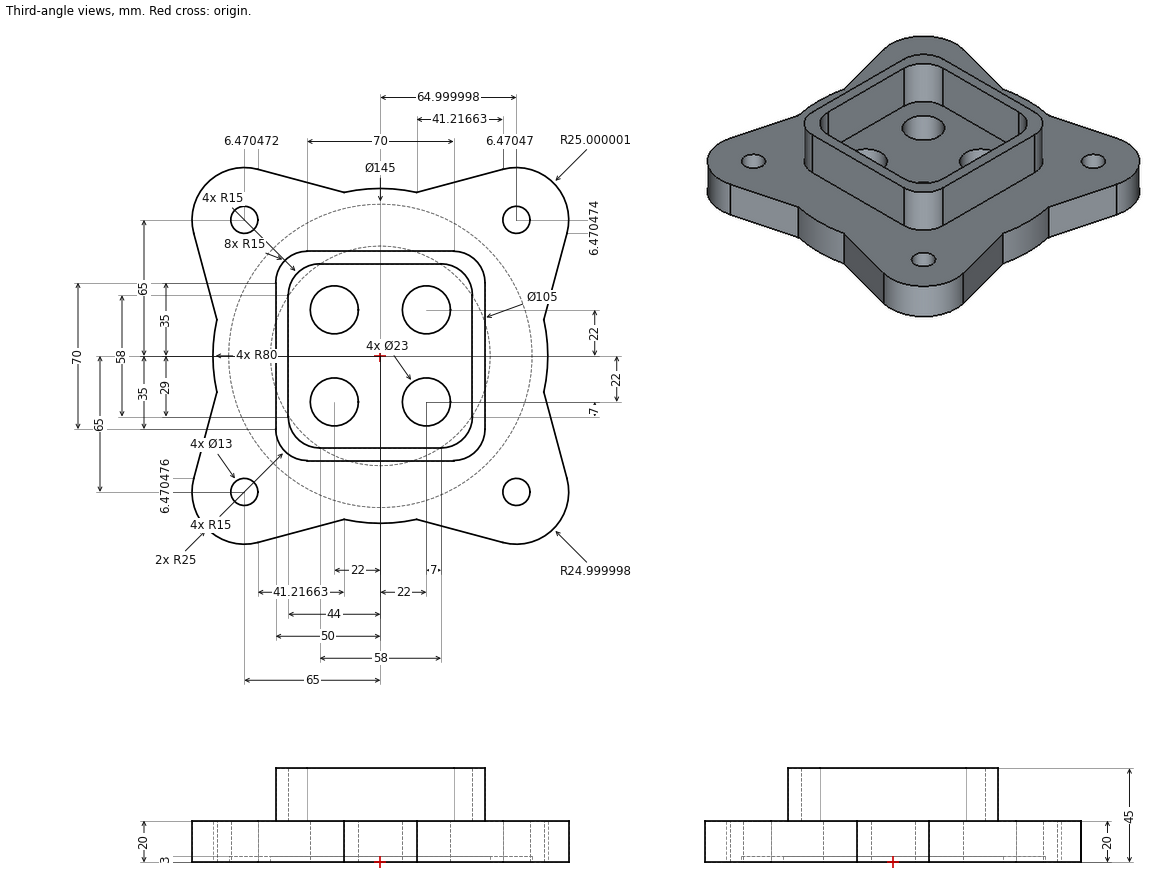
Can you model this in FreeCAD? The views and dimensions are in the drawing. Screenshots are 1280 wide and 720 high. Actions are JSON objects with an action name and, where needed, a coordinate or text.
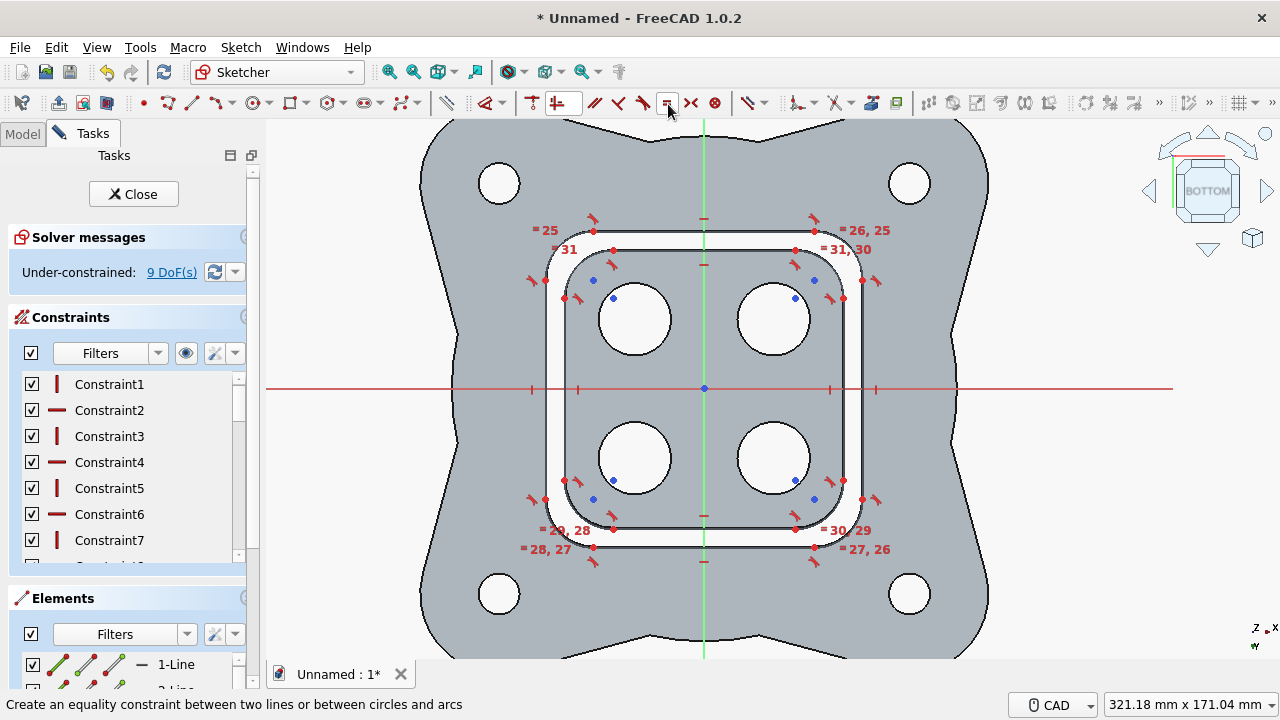
{"action": "left_click", "coordinate": [486, 104]}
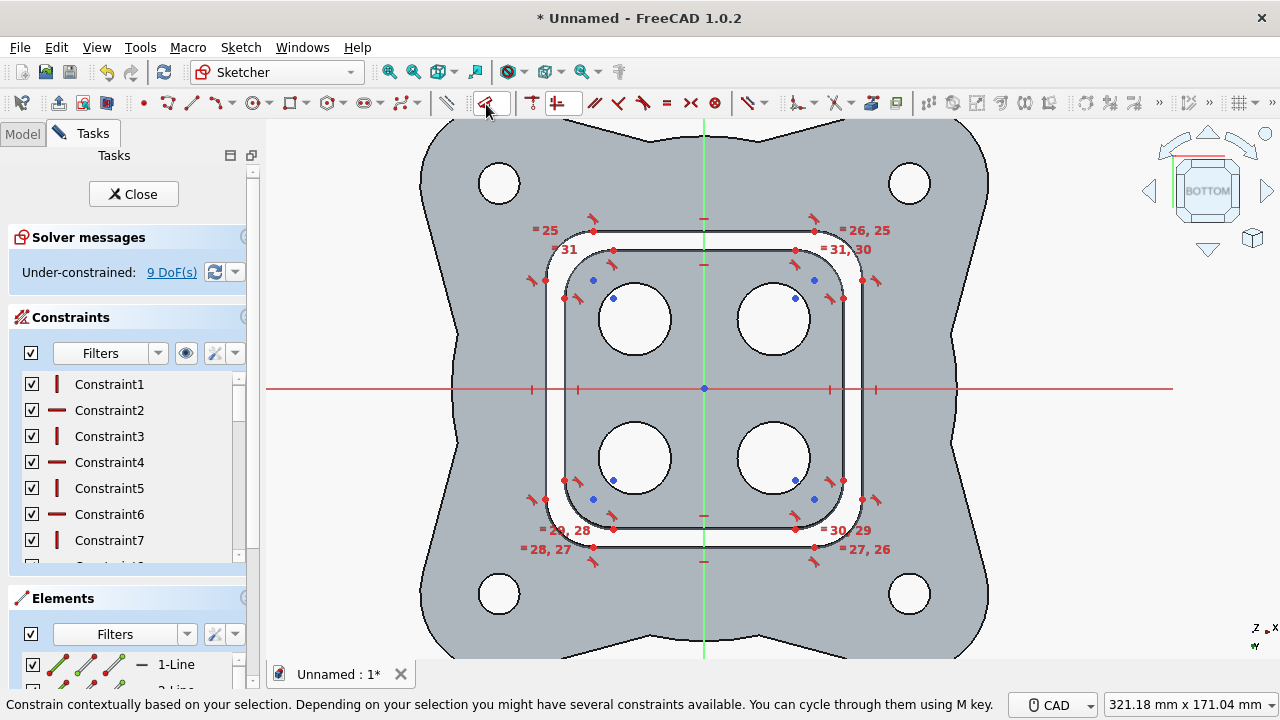
{"action": "left_click", "coordinate": [572, 237]}
{"action": "left_click", "coordinate": [557, 208]}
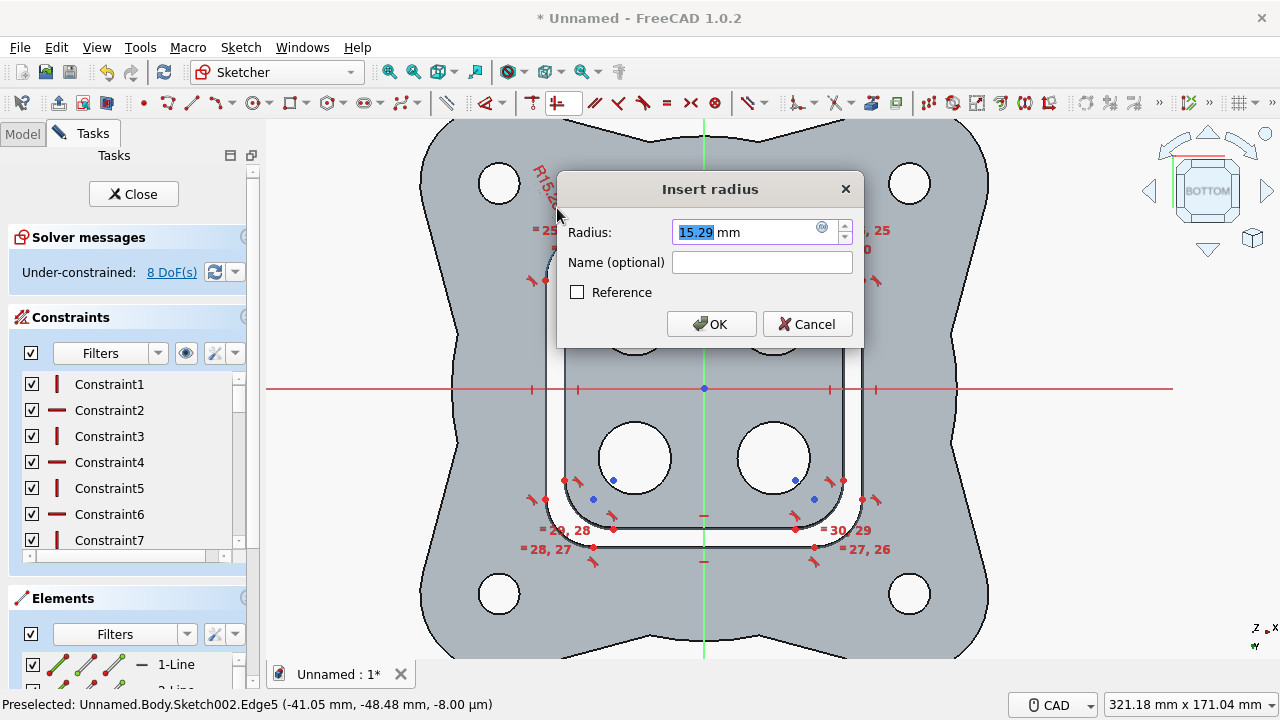
{"action": "type", "text": "15"}
{"action": "key", "text": "Return"}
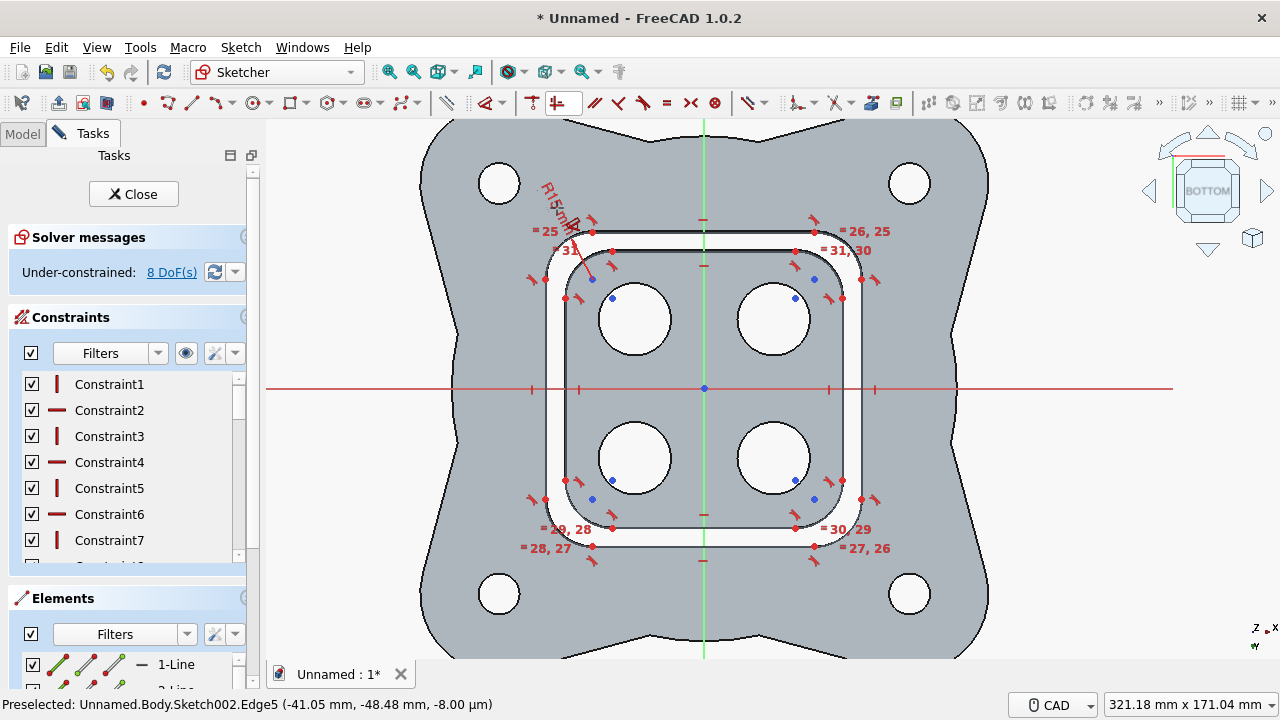
{"action": "left_click", "coordinate": [546, 434]}
{"action": "left_click", "coordinate": [512, 339]}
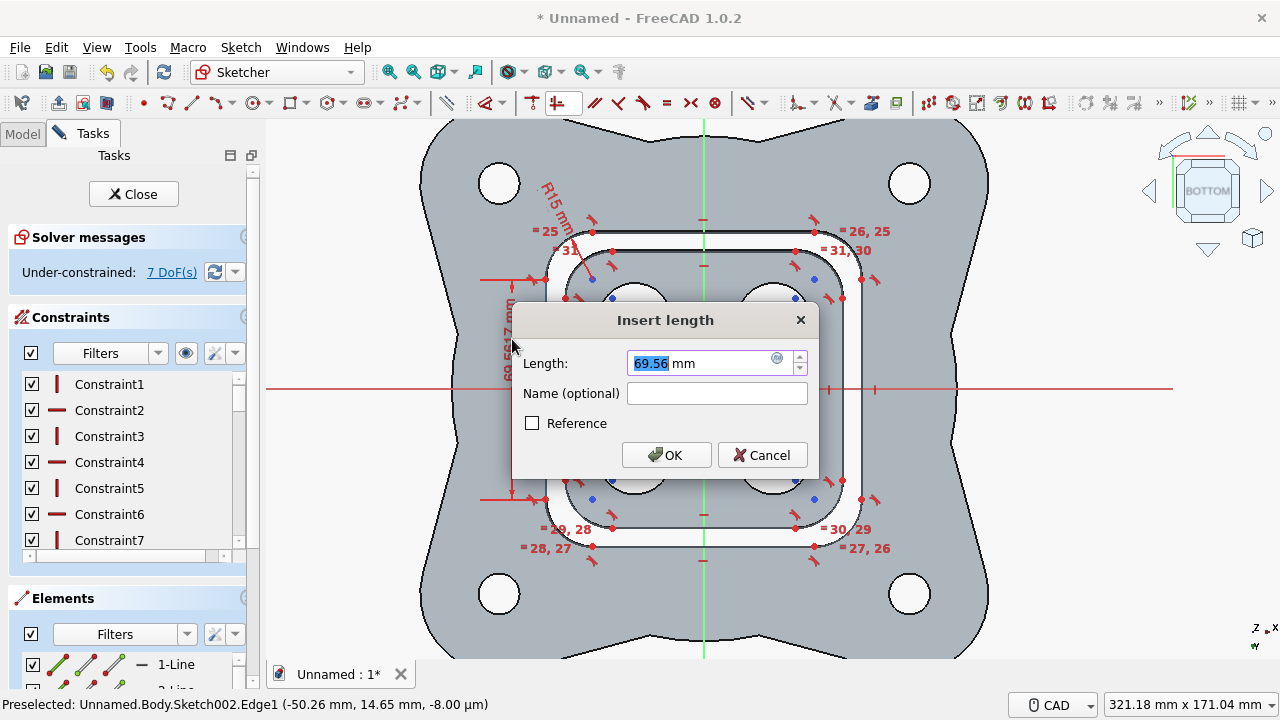
{"action": "type", "text": "70"}
{"action": "key", "text": "Return"}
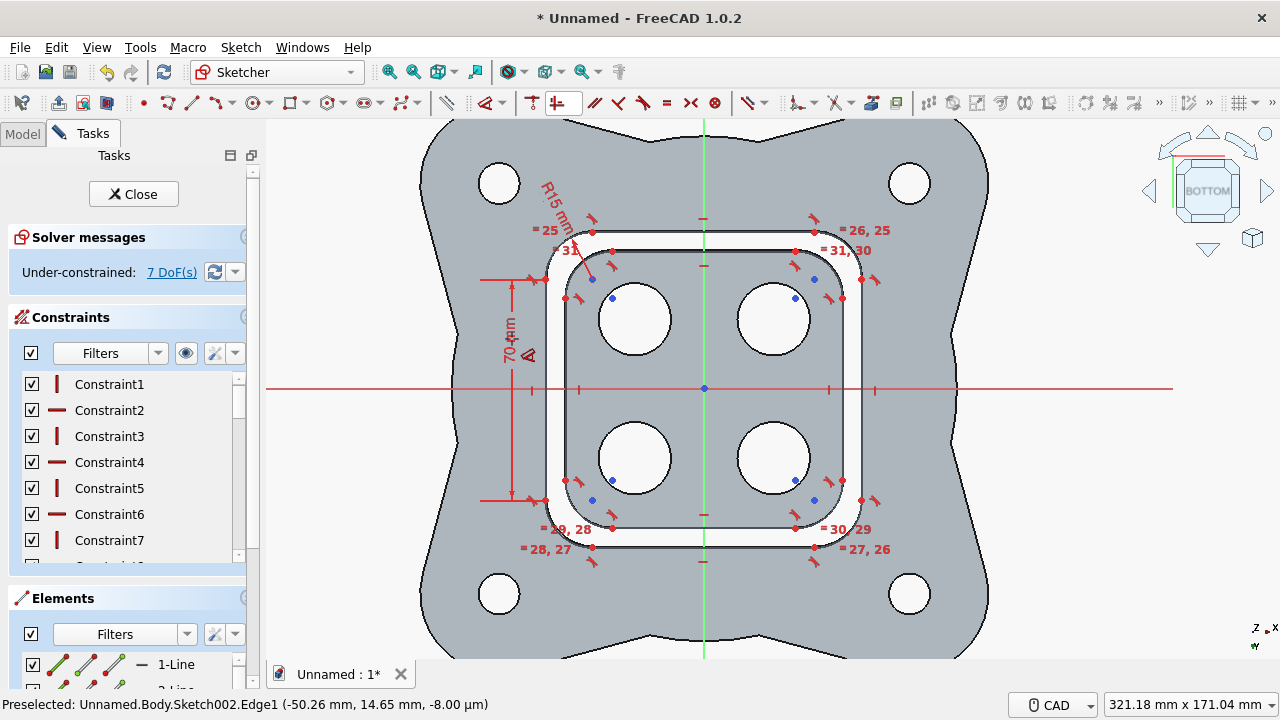
{"action": "left_click", "coordinate": [659, 232]}
{"action": "left_click", "coordinate": [653, 198]}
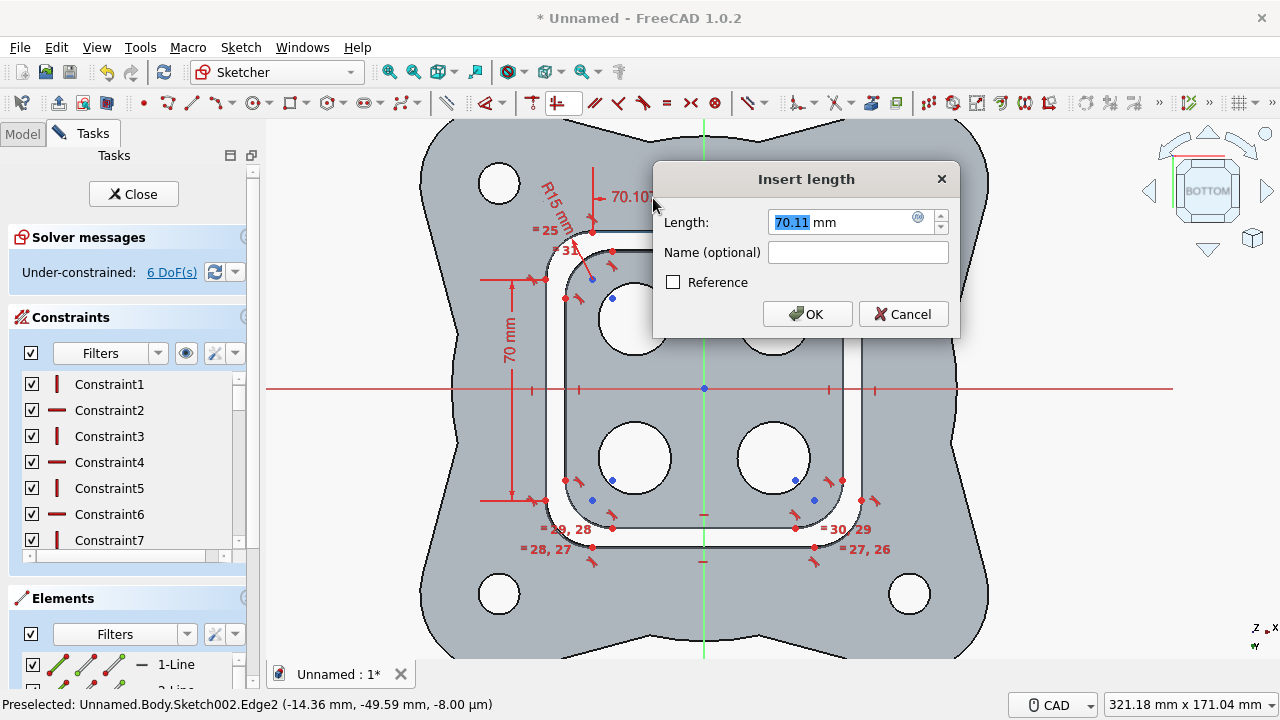
{"action": "type", "text": "70"}
{"action": "key", "text": "Return"}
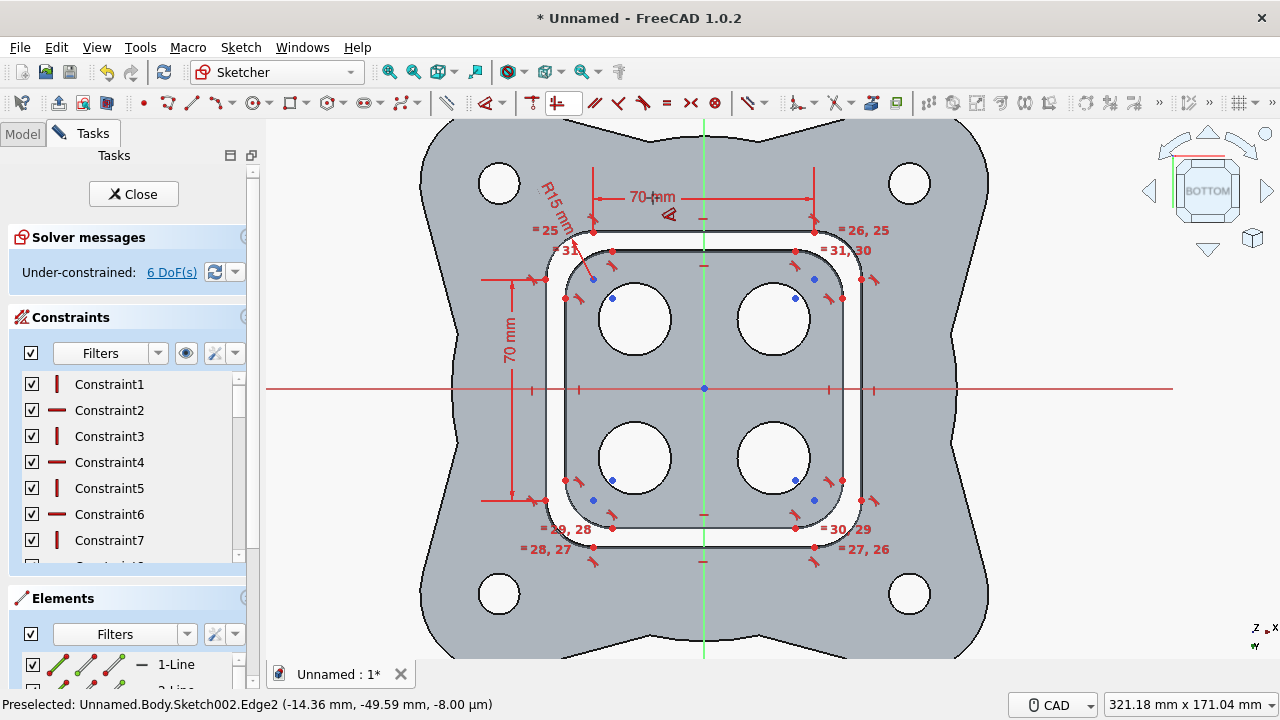
{"action": "left_click", "coordinate": [566, 354]}
{"action": "left_click", "coordinate": [532, 432]}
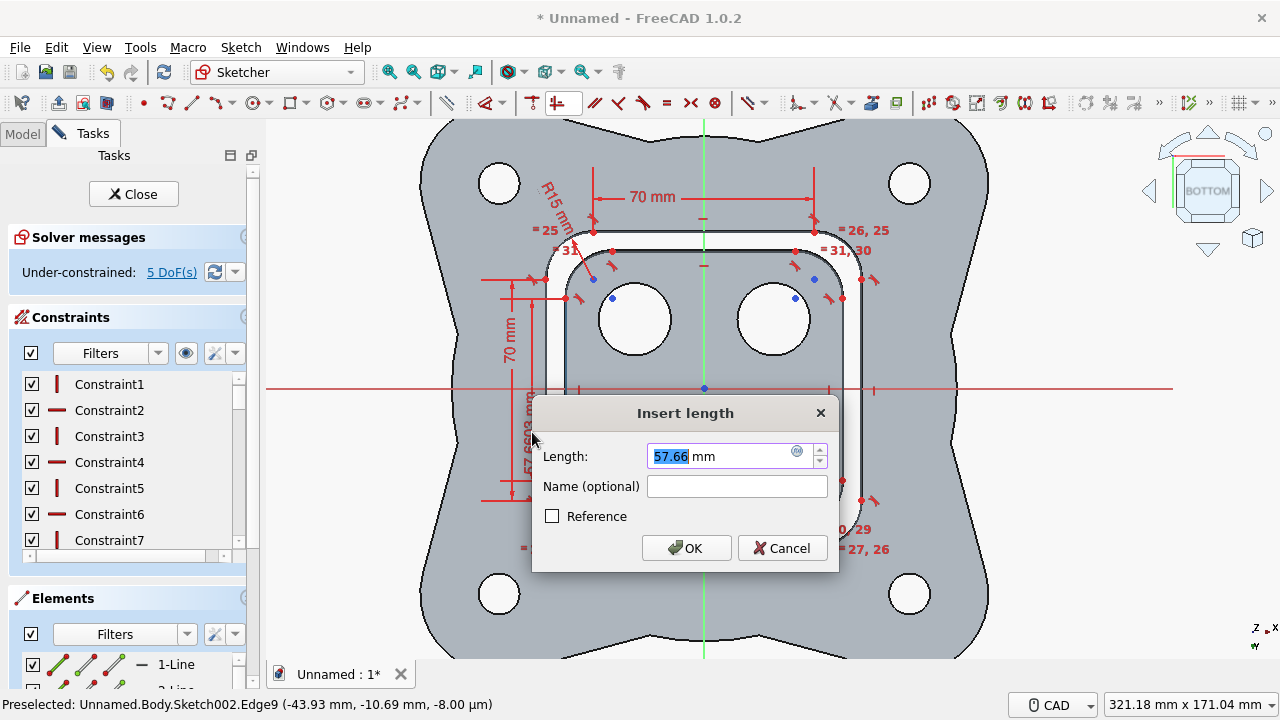
{"action": "type", "text": "58"}
{"action": "key", "text": "Return"}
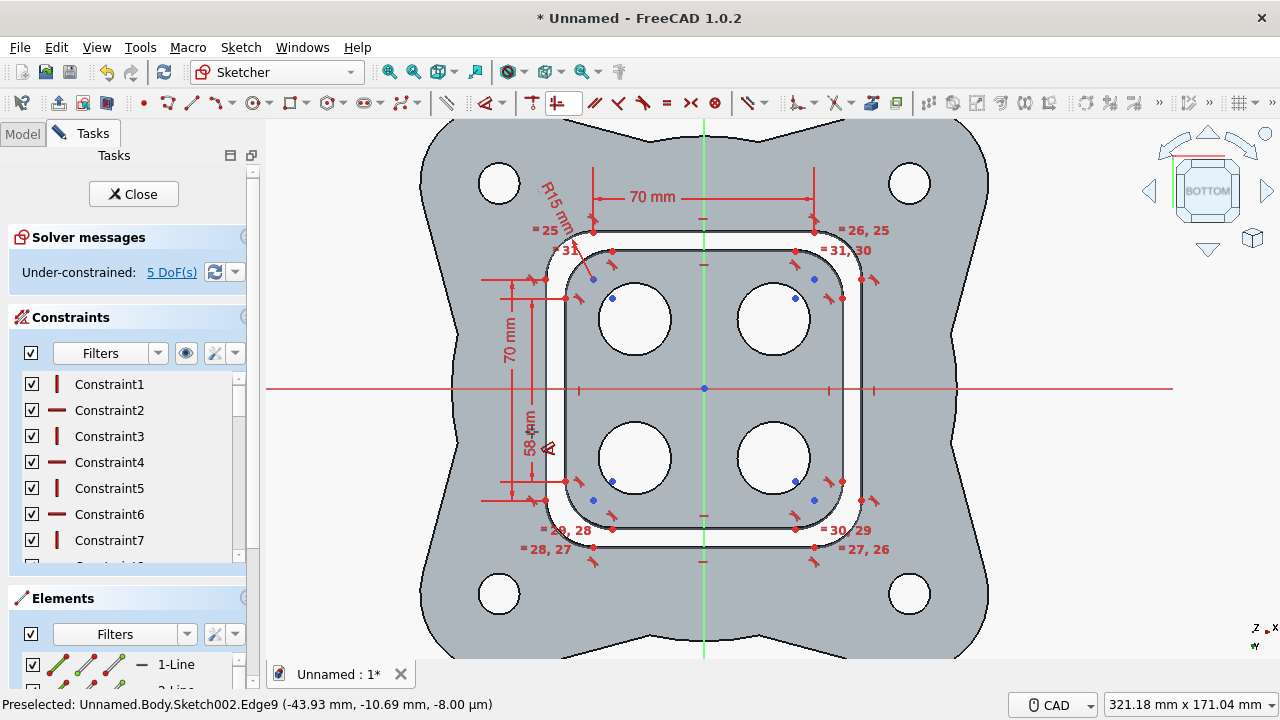
{"action": "left_click", "coordinate": [668, 529]}
{"action": "left_click", "coordinate": [662, 563]}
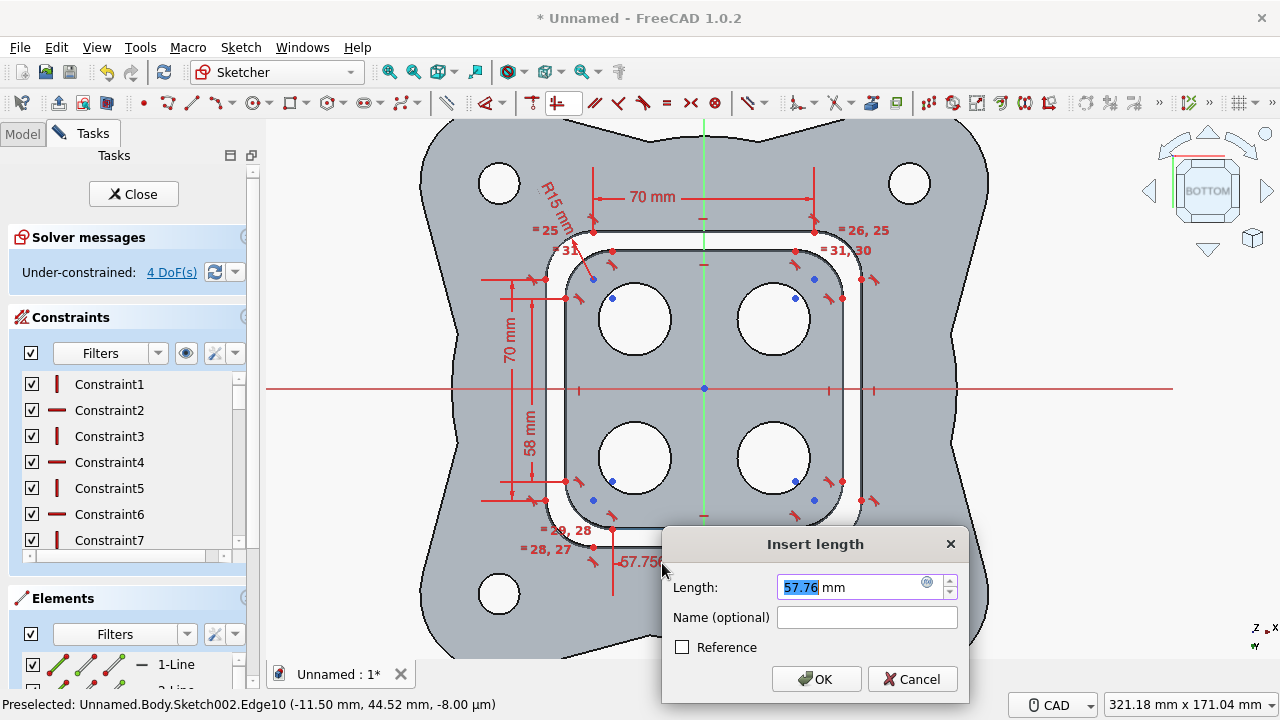
{"action": "type", "text": "58"}
{"action": "key", "text": "Return"}